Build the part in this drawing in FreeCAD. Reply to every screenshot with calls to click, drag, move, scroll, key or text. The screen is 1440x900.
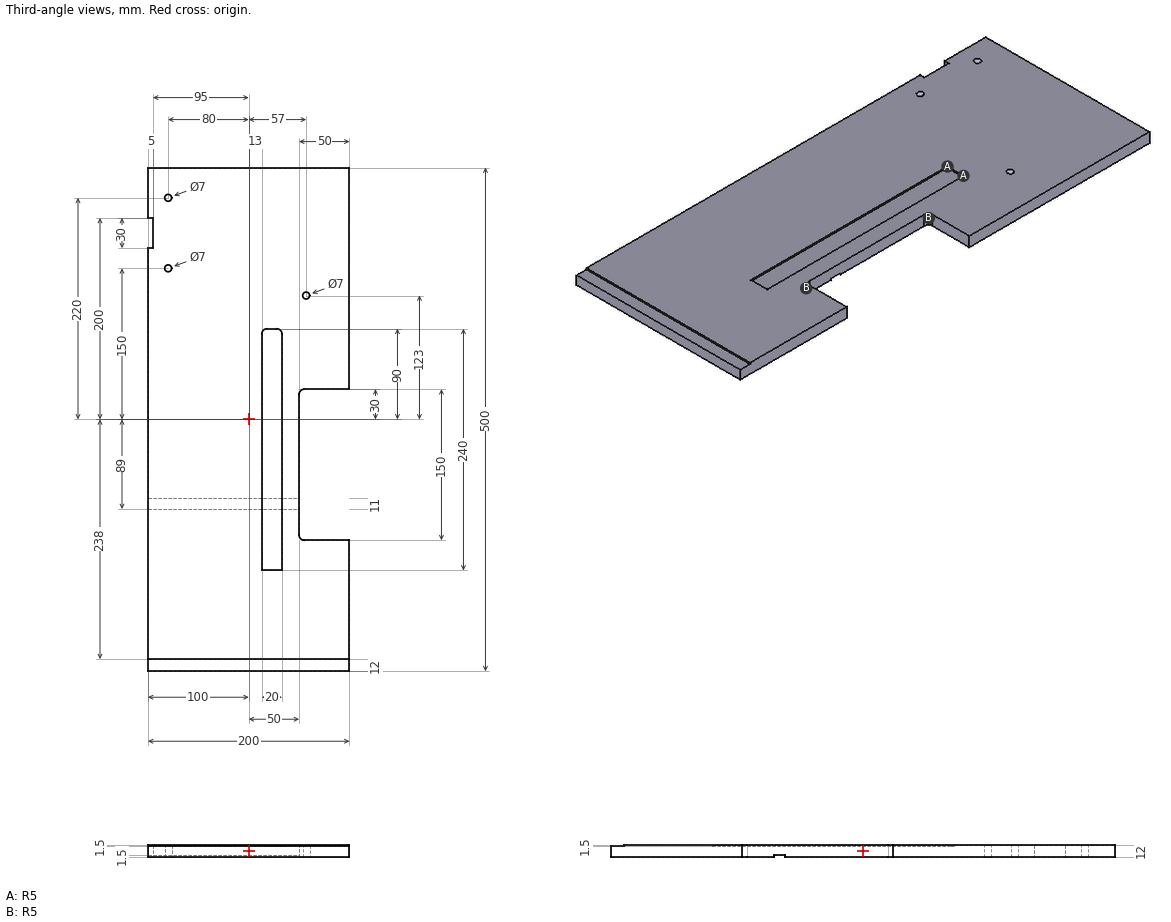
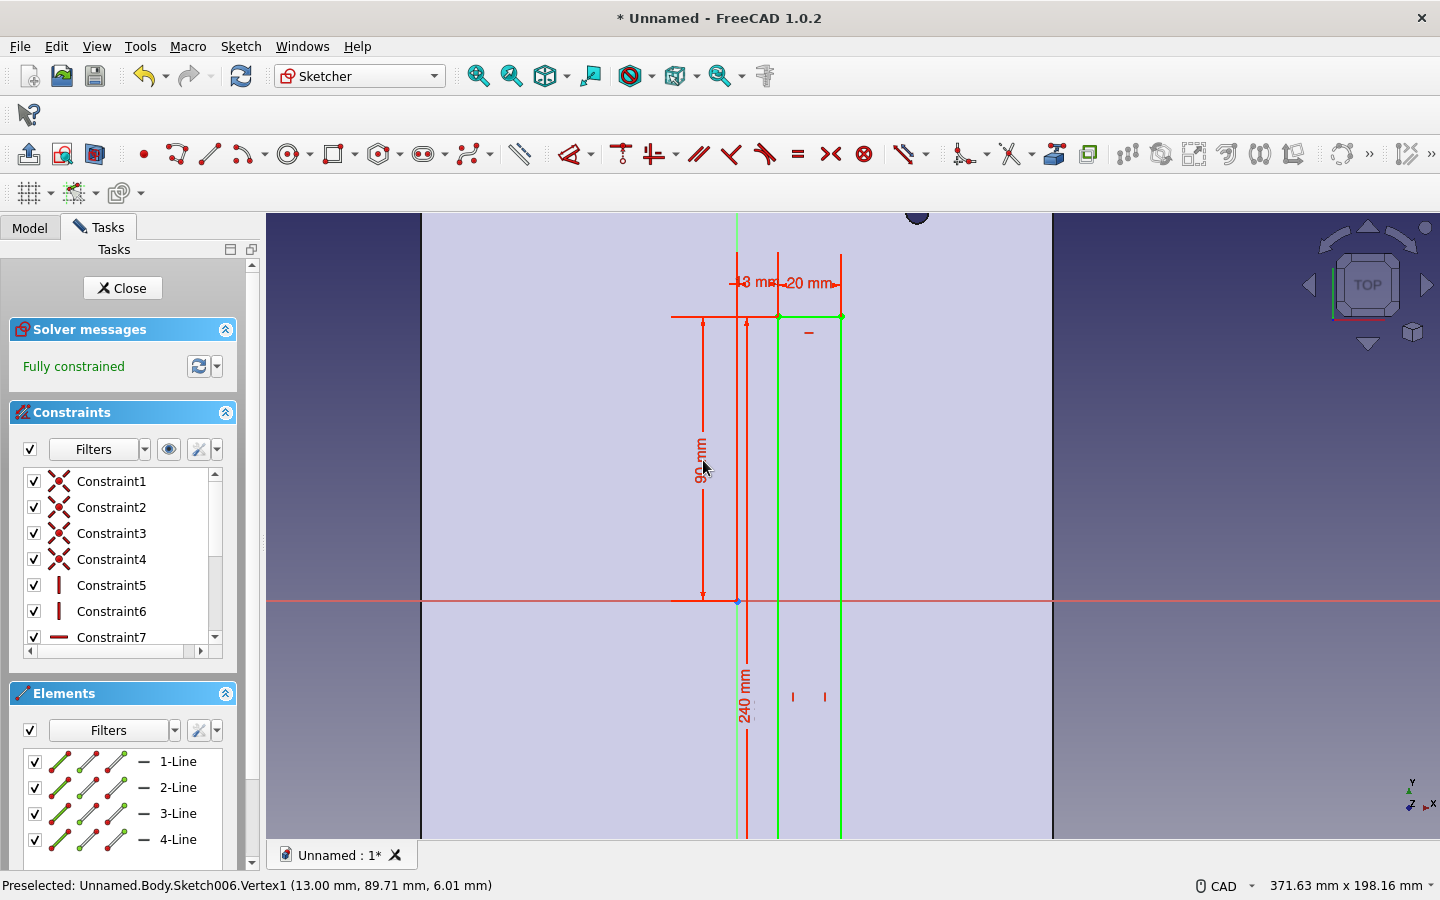
click(123, 288)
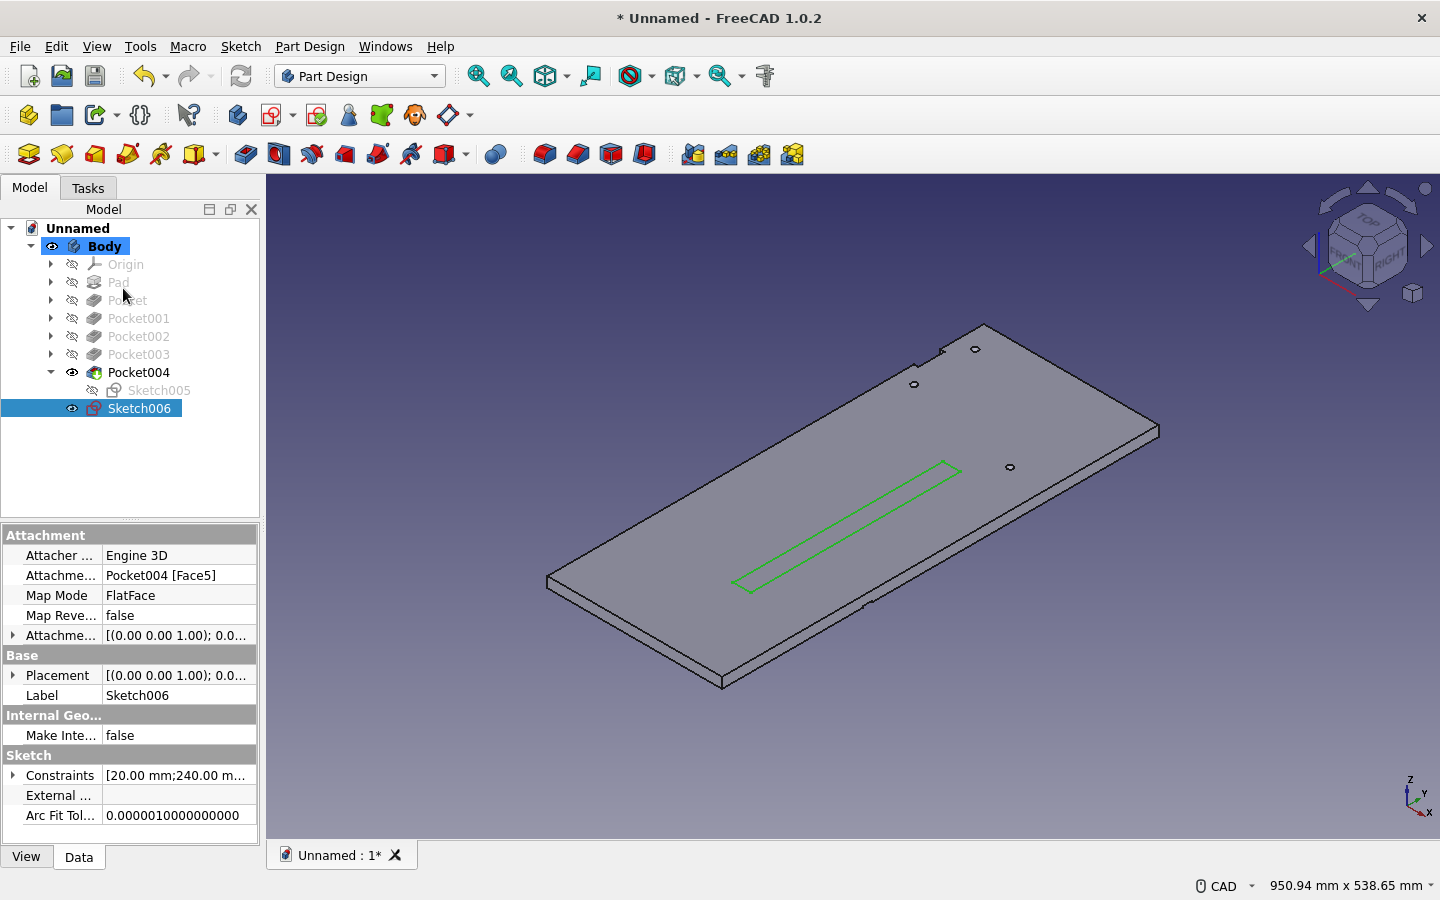
click(246, 154)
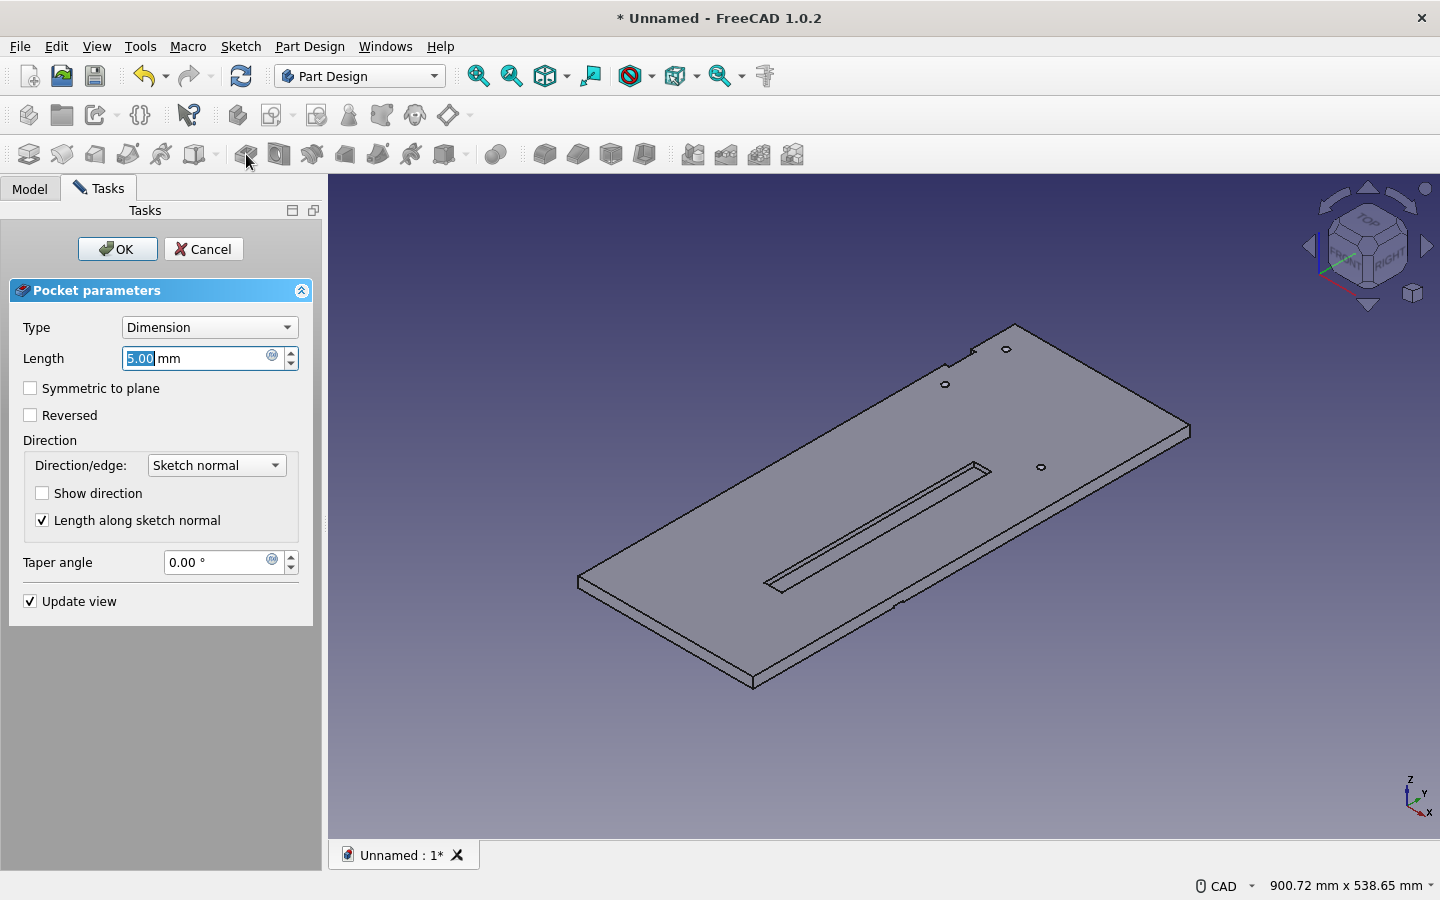
text(1.5)
key(Tab)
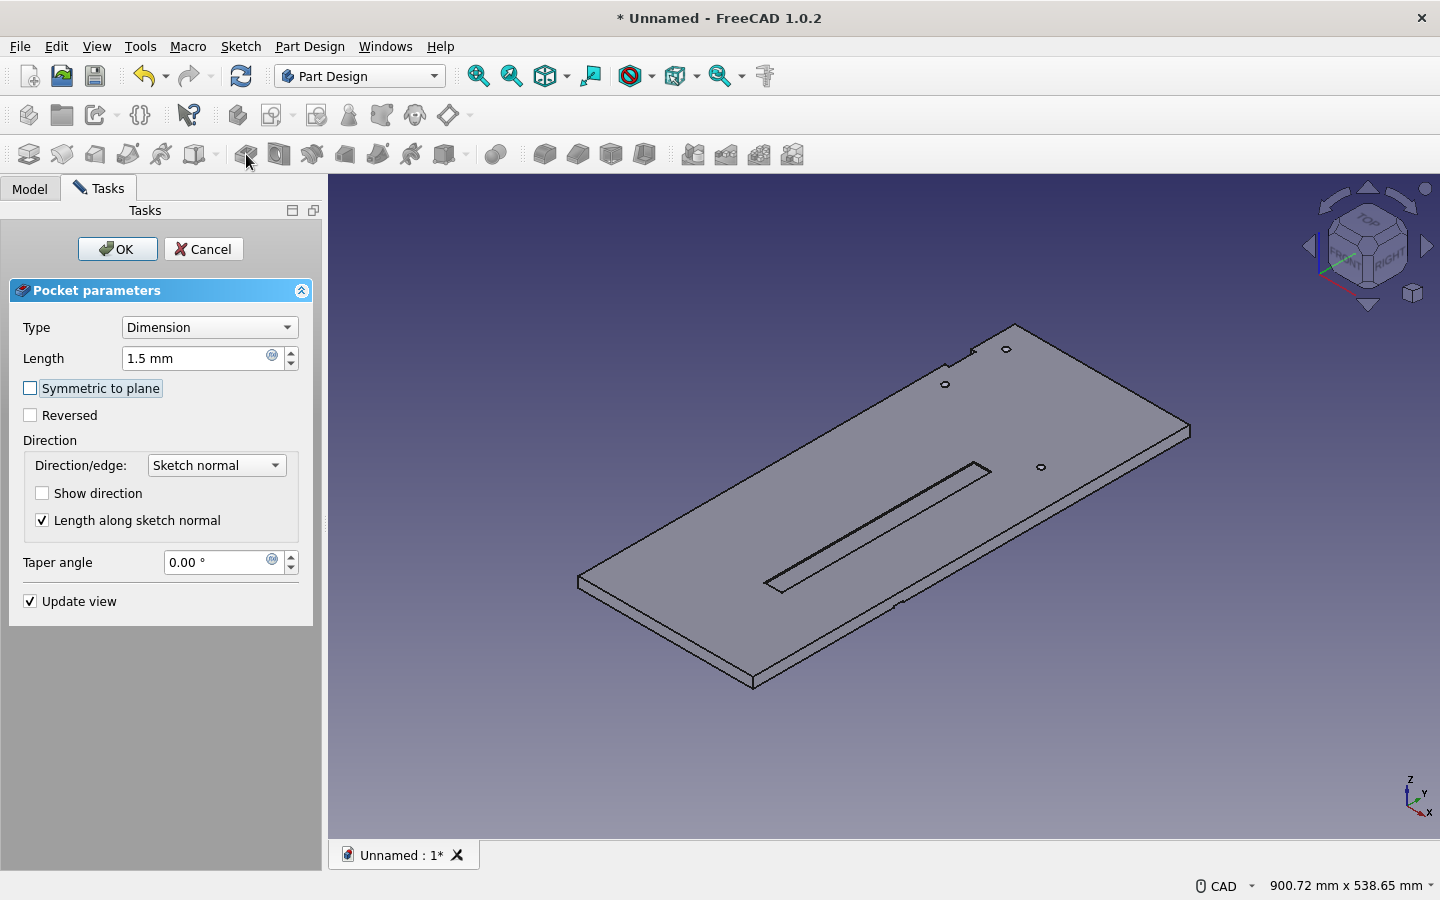
click(118, 249)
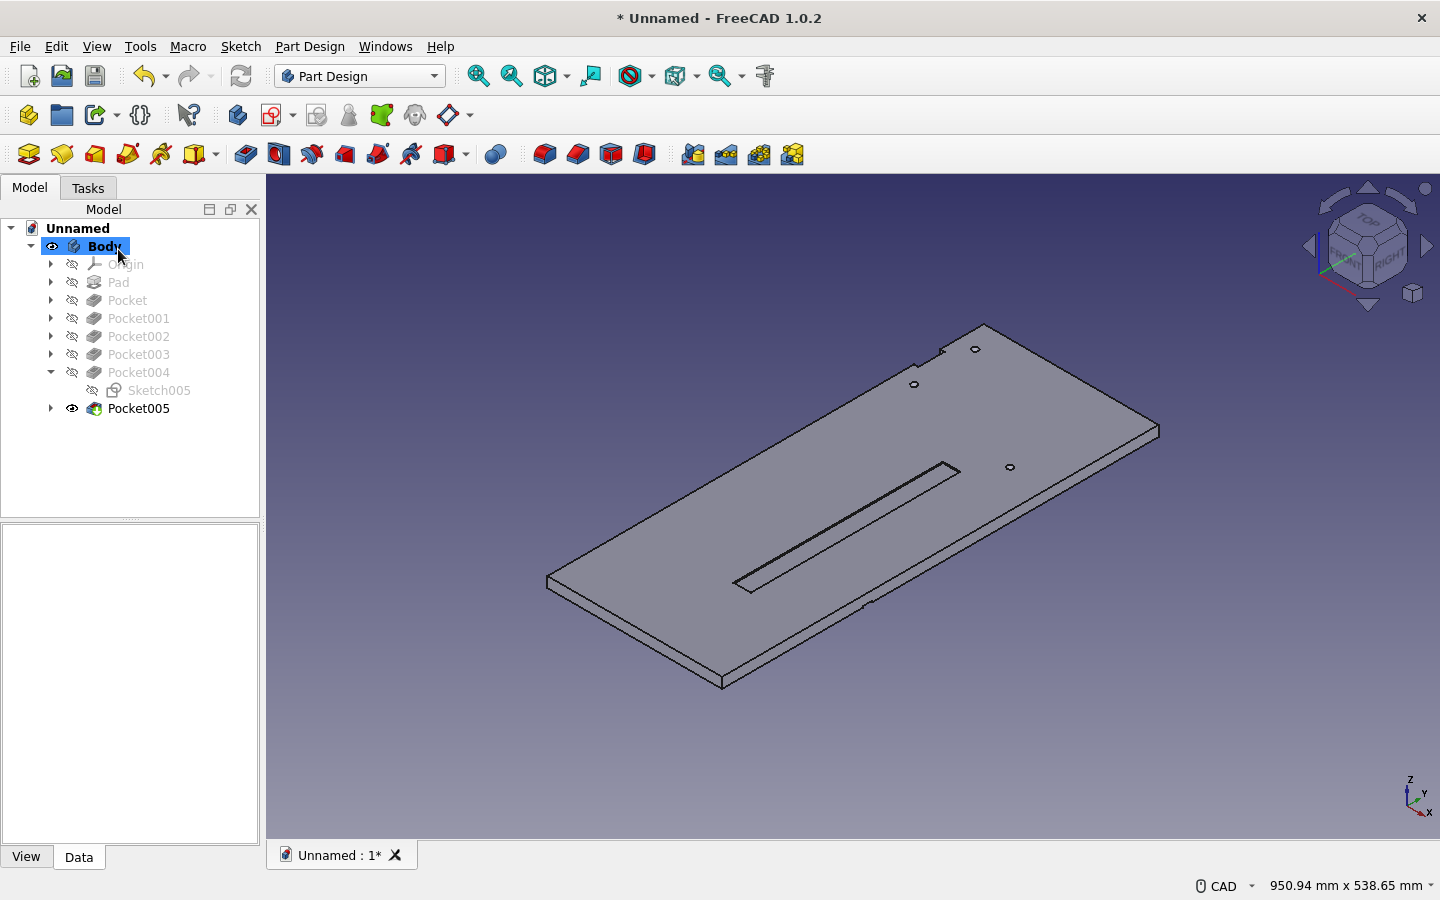
scroll(960, 471, up, 15)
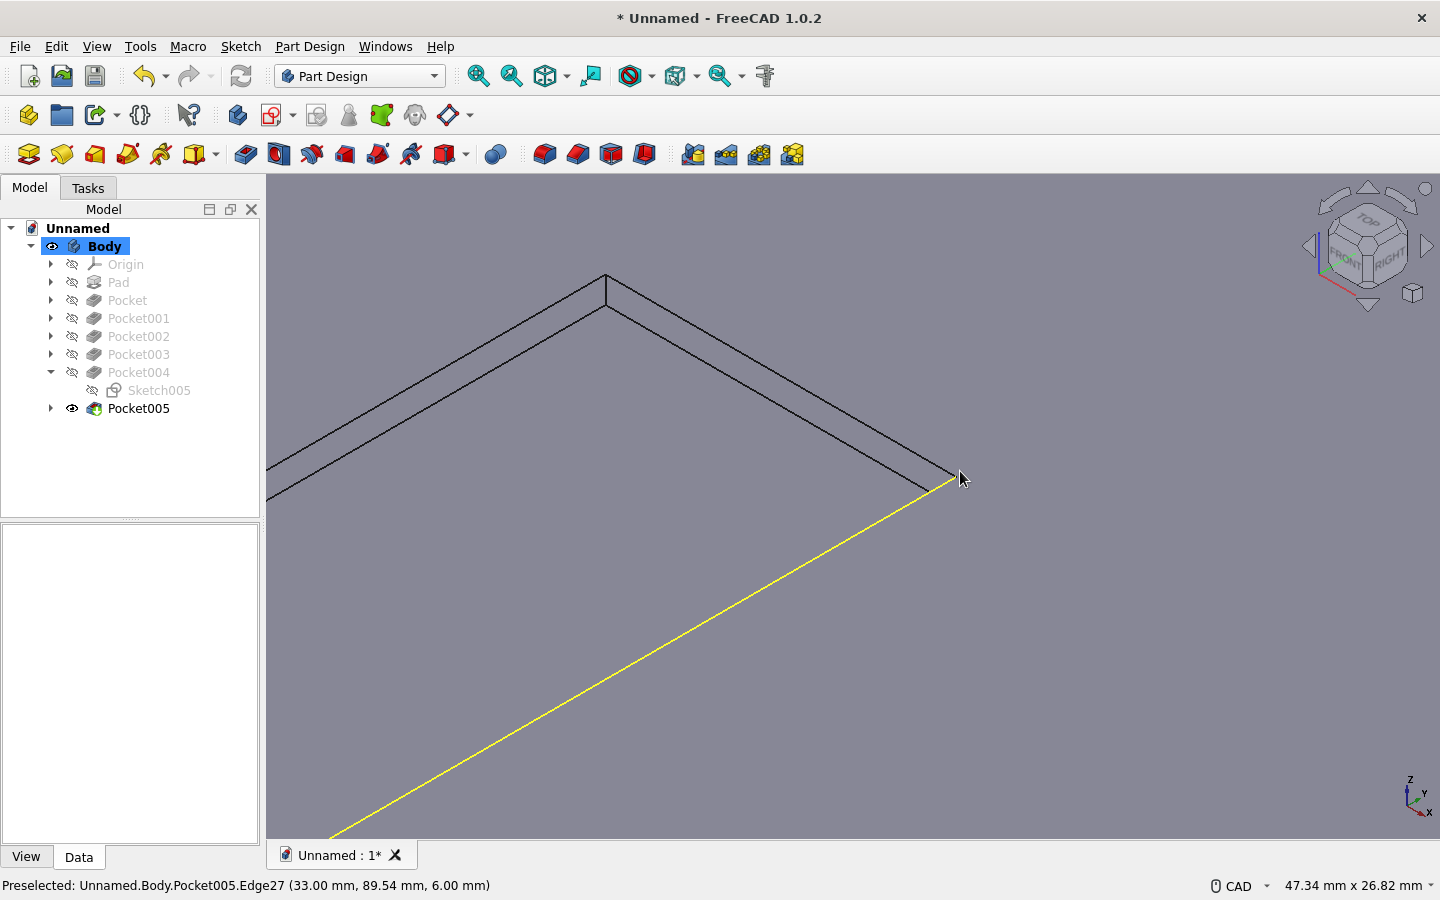
click(479, 76)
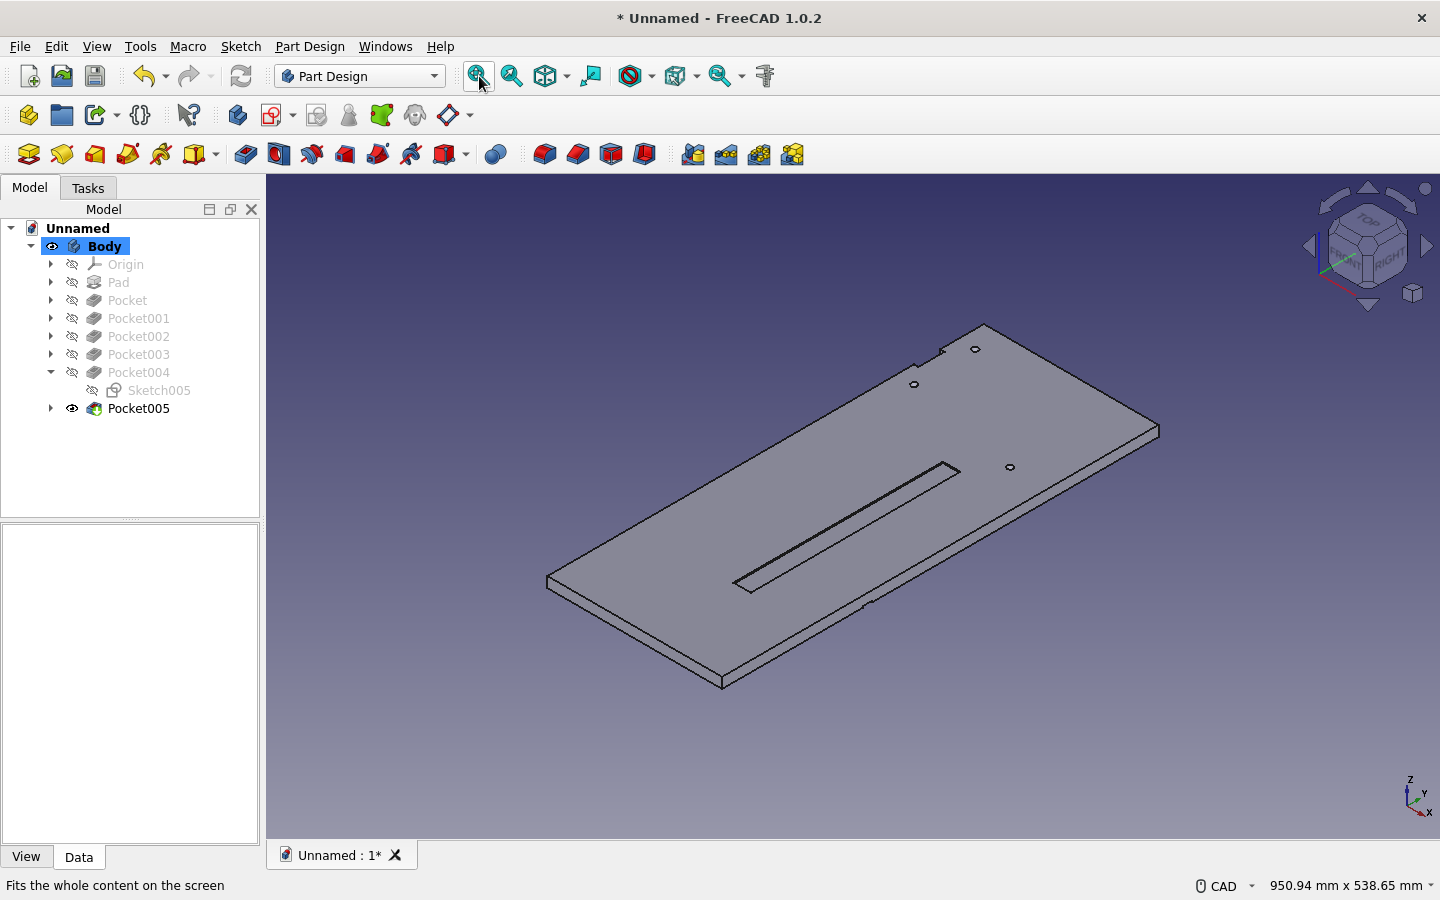
key(2)